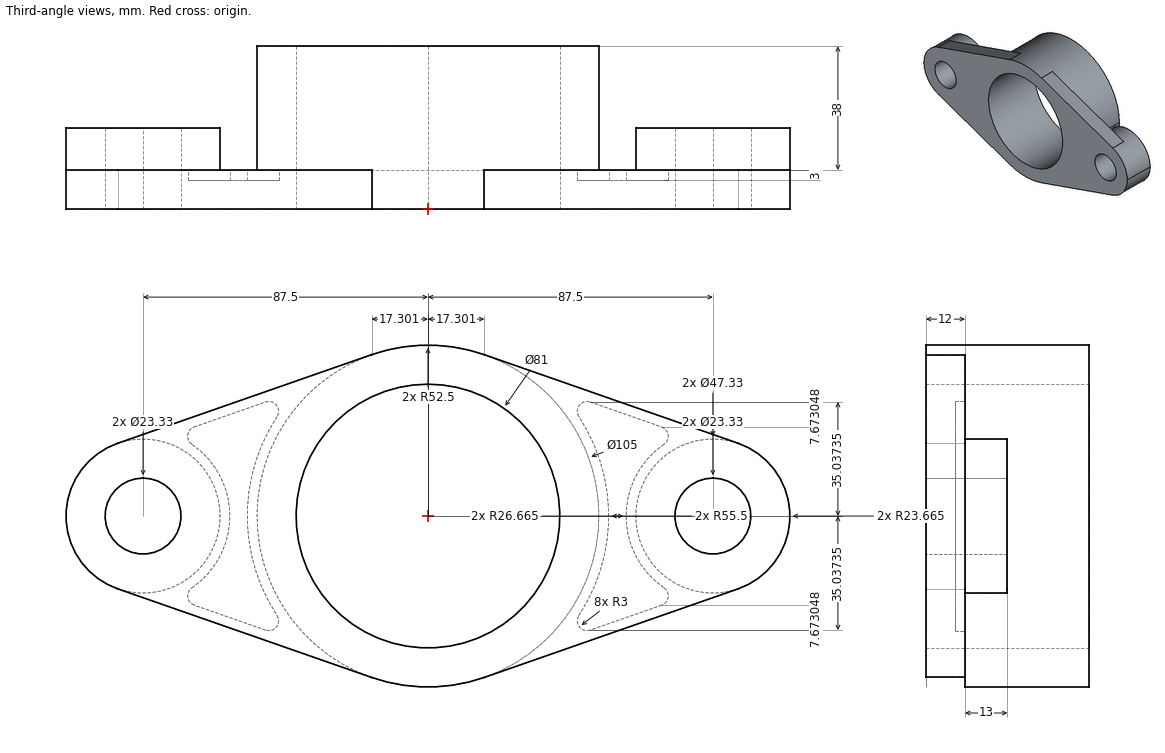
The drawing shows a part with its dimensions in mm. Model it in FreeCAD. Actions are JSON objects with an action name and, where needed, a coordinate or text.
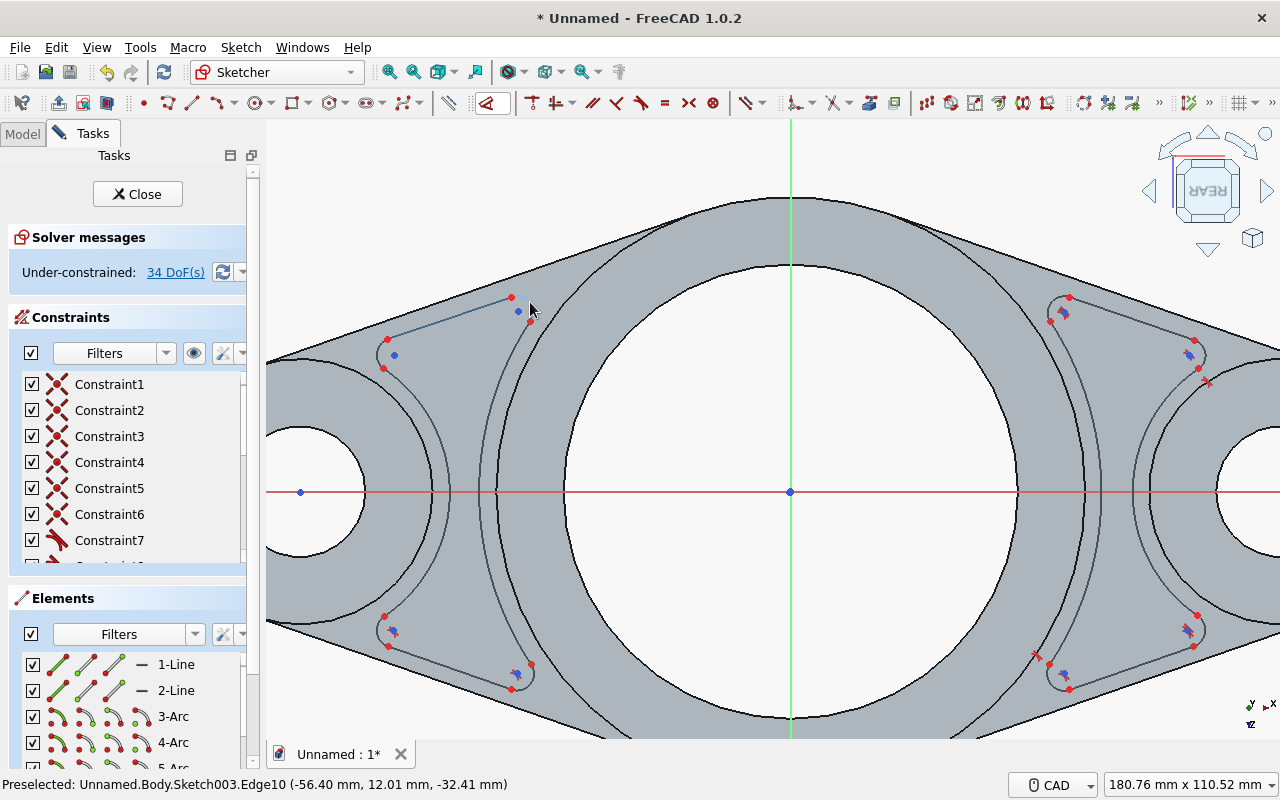
{"action": "left_click", "coordinate": [530, 302]}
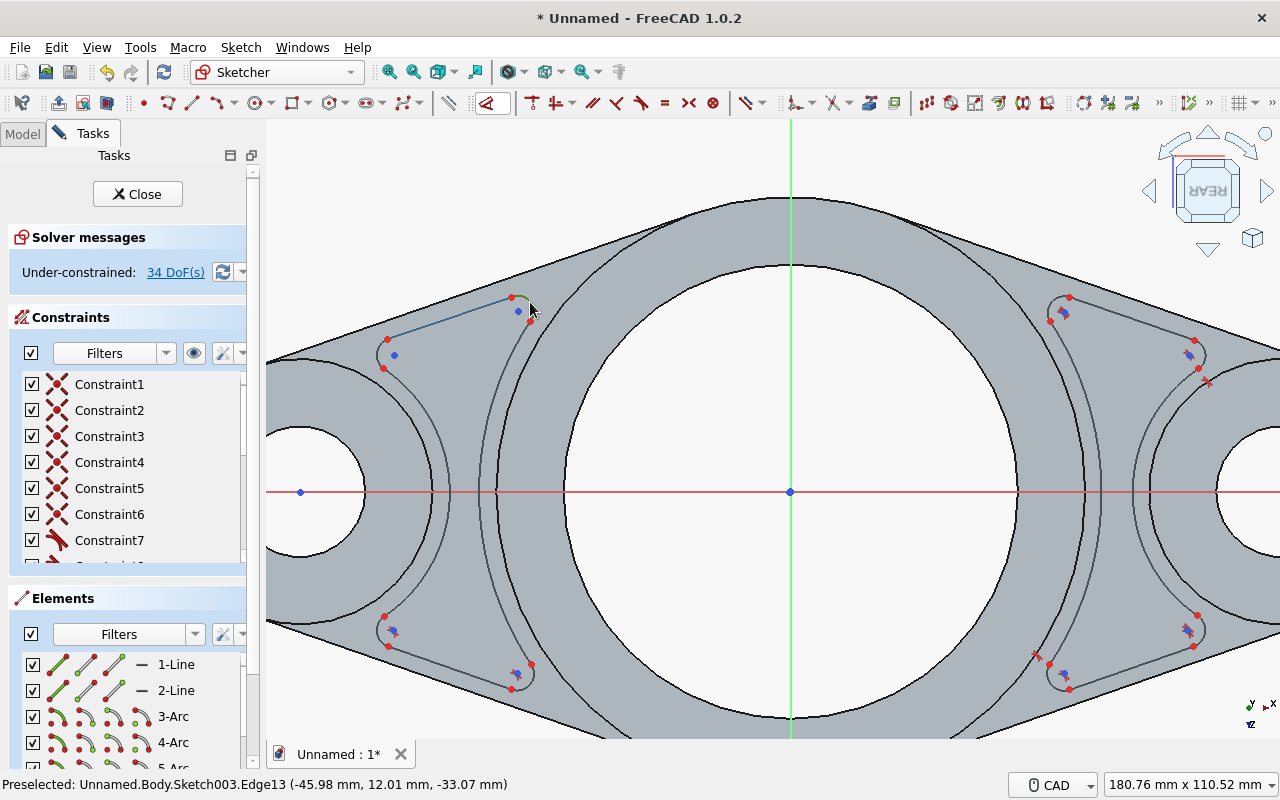
{"action": "left_click", "coordinate": [642, 104]}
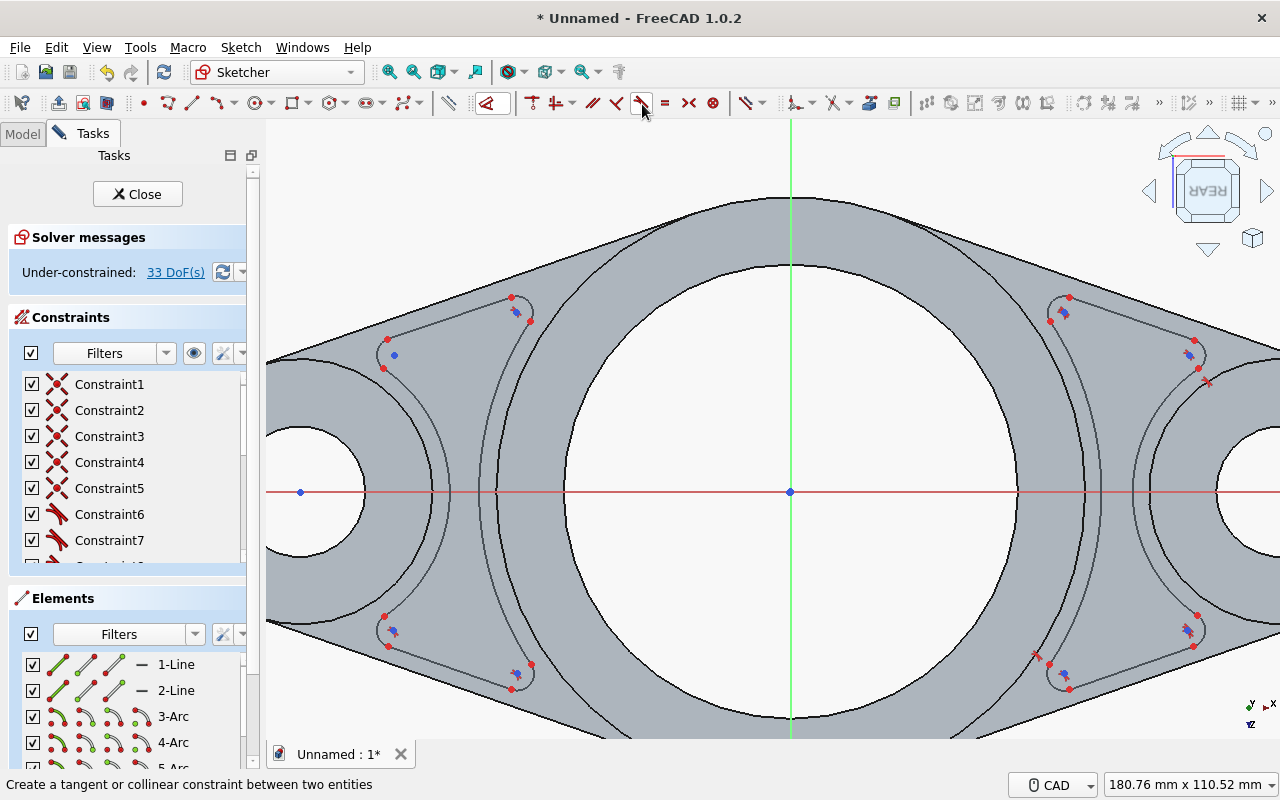
{"action": "left_click", "coordinate": [475, 310]}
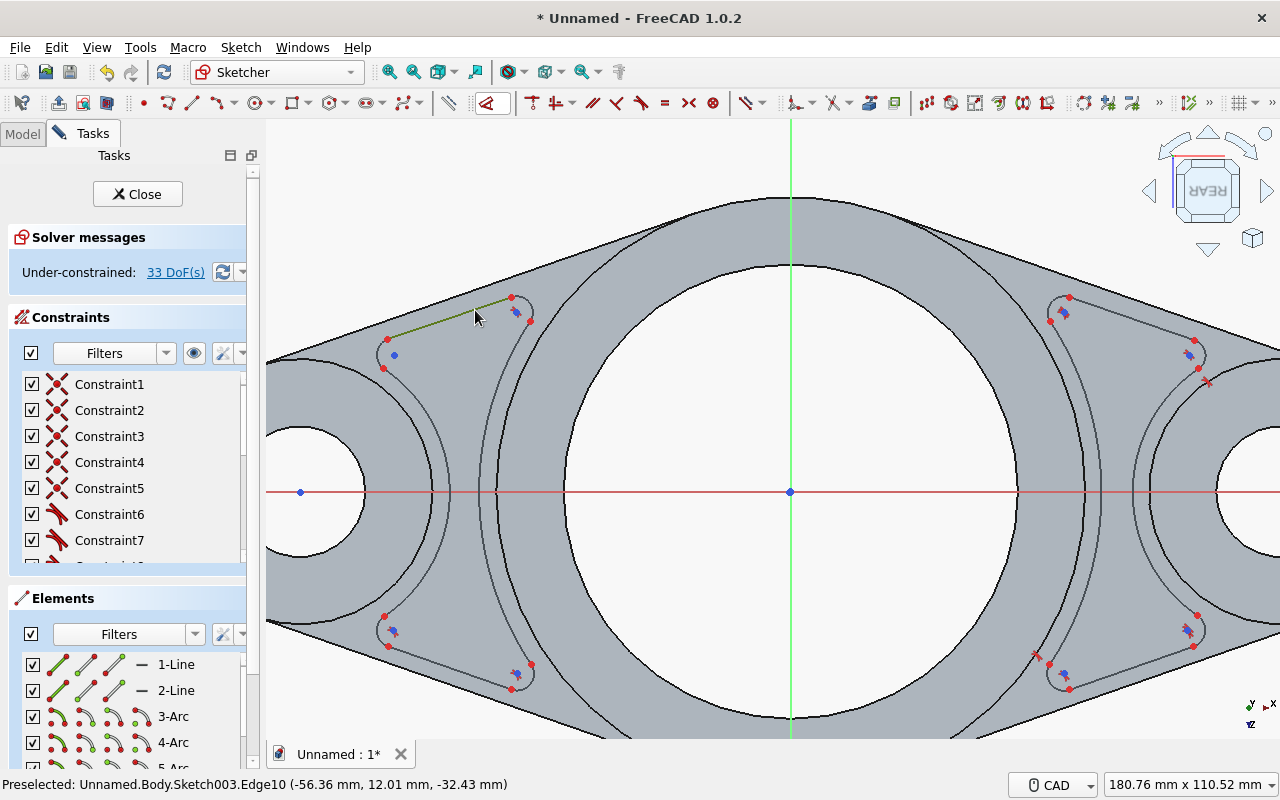
{"action": "scroll", "coordinate": [380, 346], "scroll_direction": "up", "scroll_amount": 2}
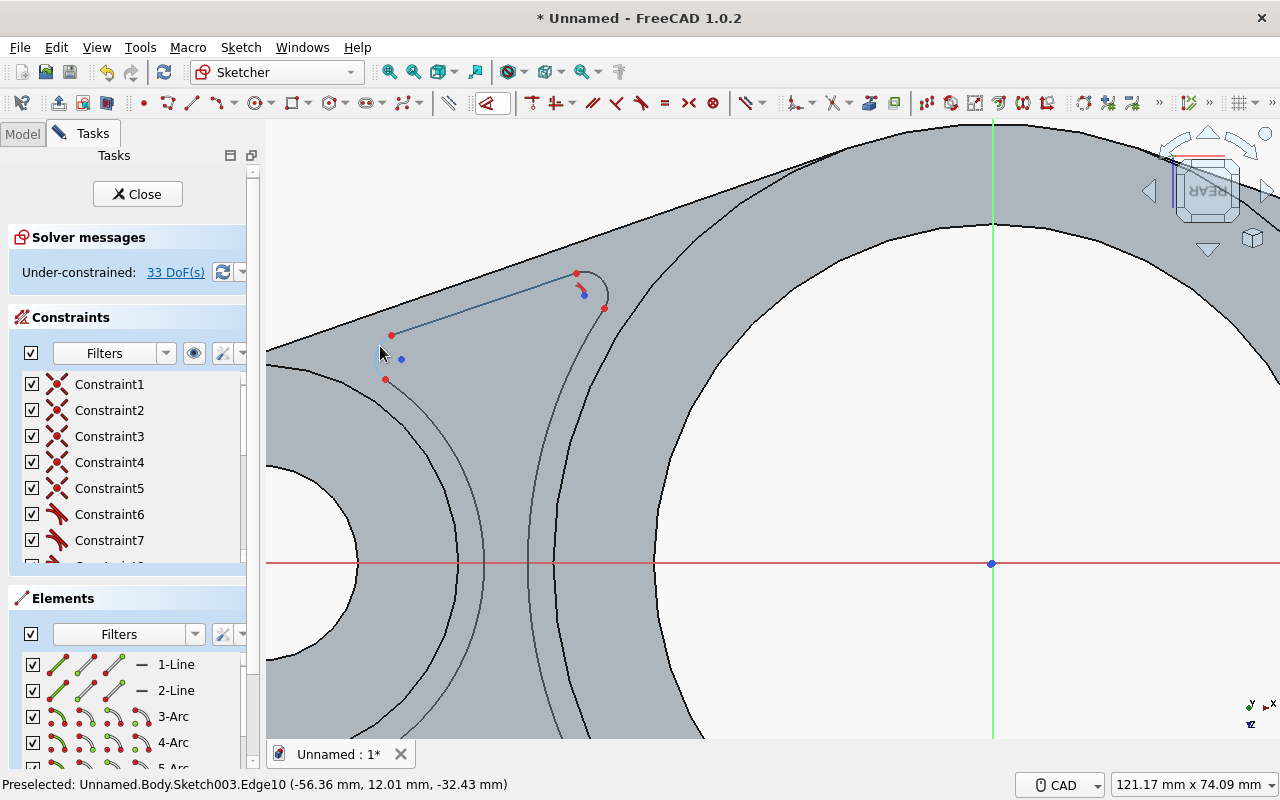
{"action": "left_click", "coordinate": [379, 346]}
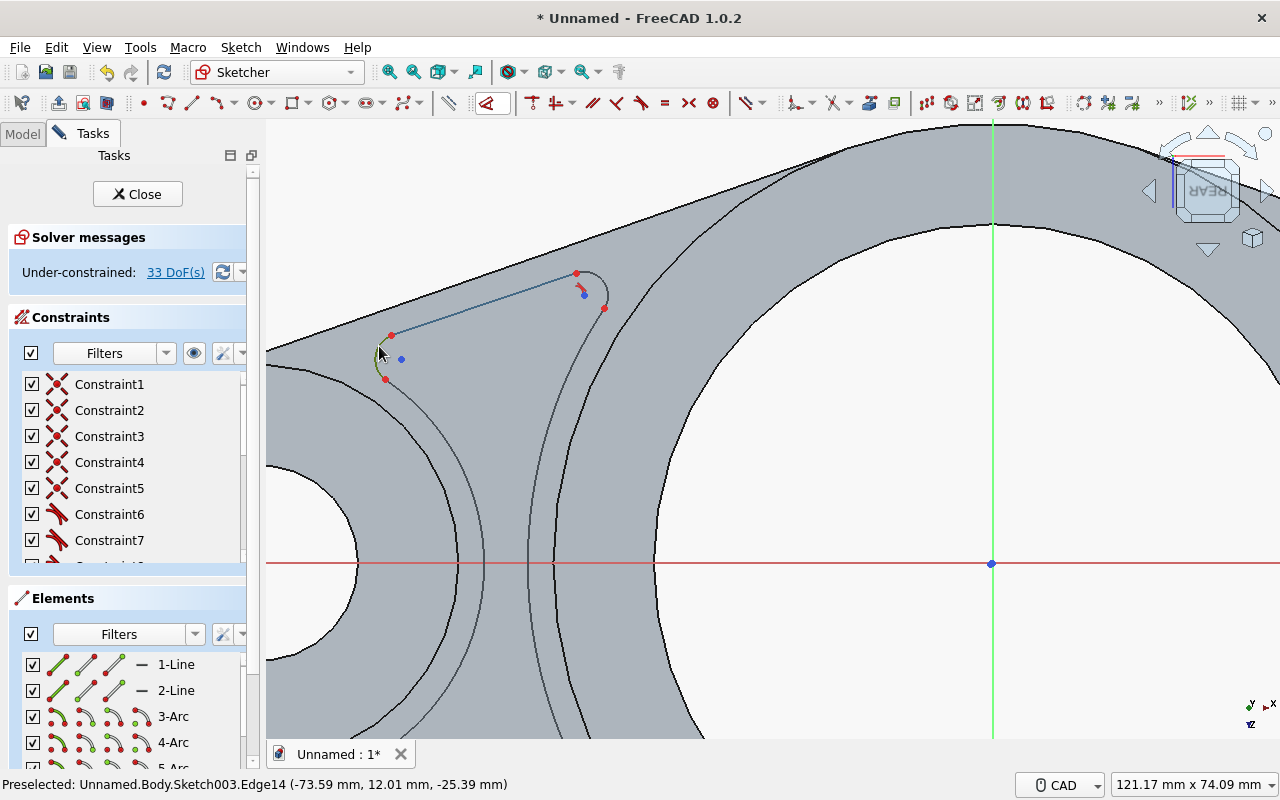
{"action": "left_click", "coordinate": [642, 104]}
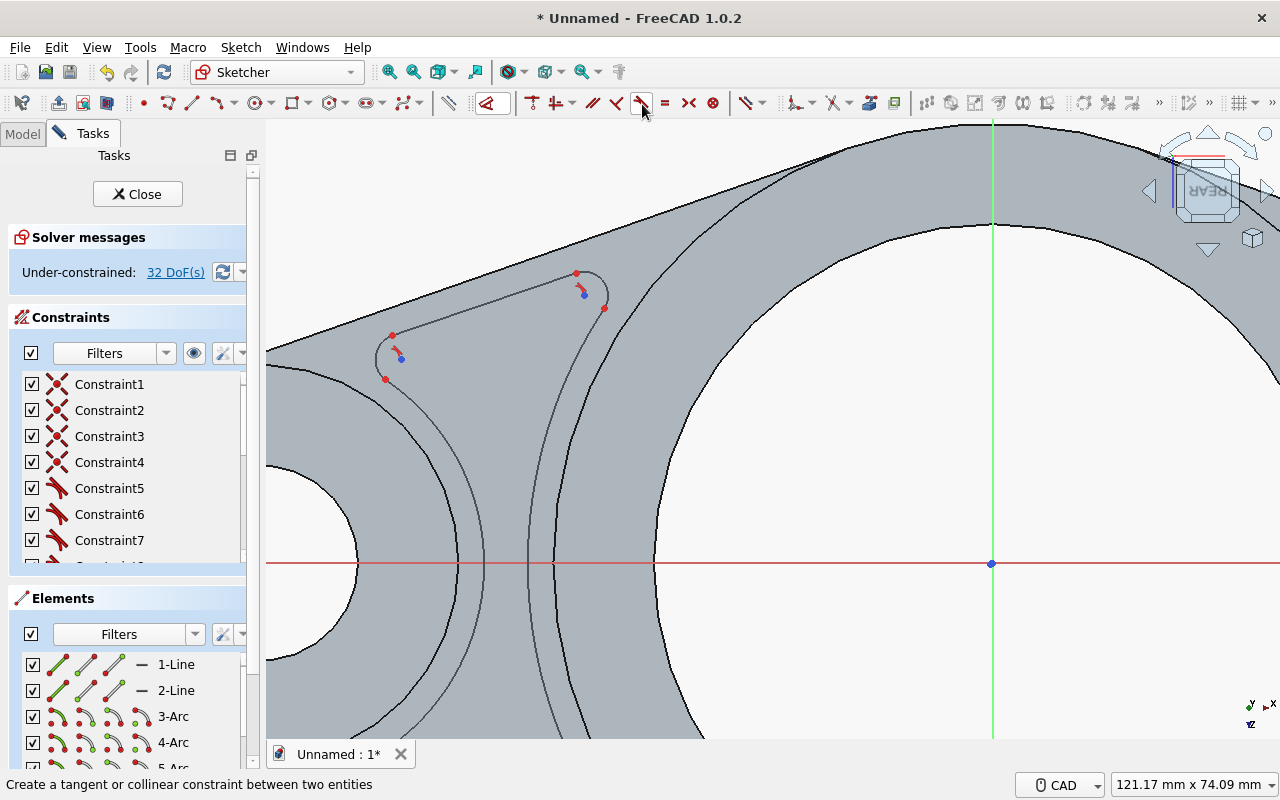
{"action": "scroll", "coordinate": [469, 320], "scroll_direction": "down", "scroll_amount": 4}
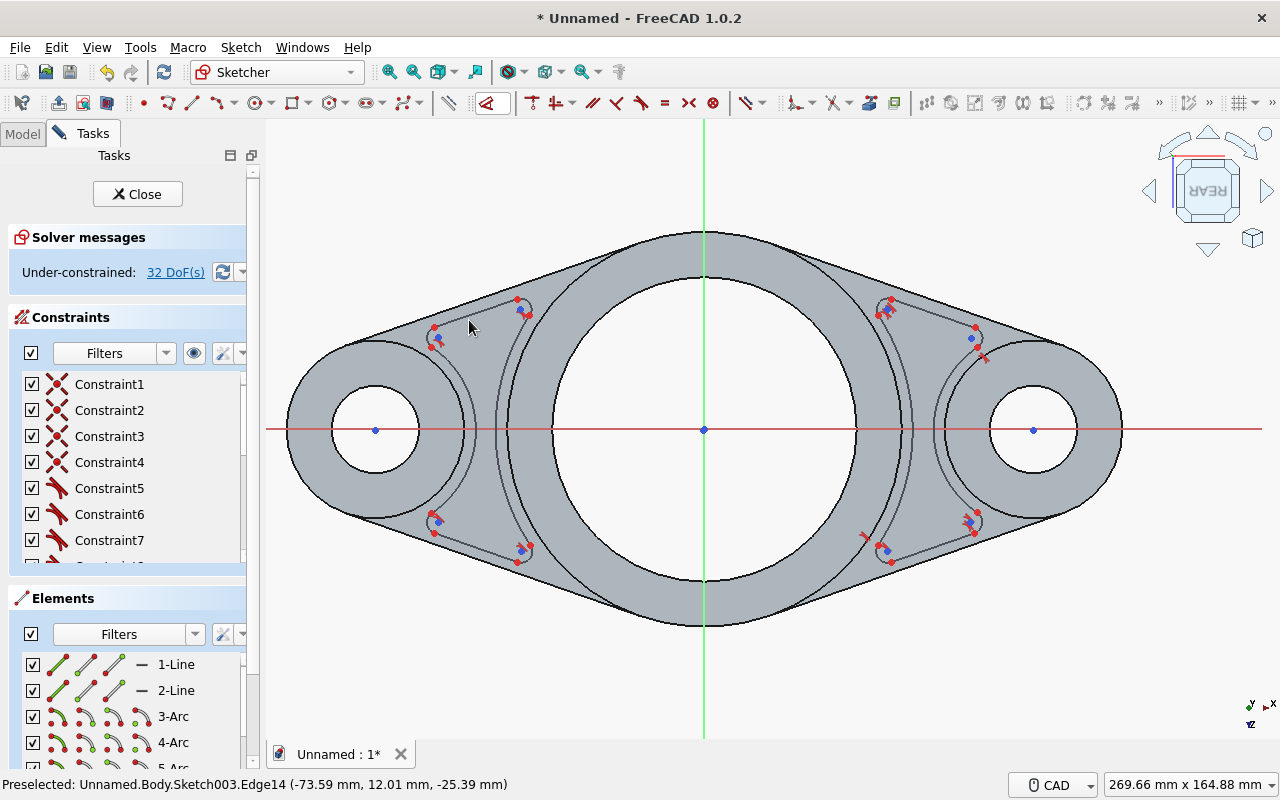
{"action": "scroll", "coordinate": [526, 562], "scroll_direction": "up", "scroll_amount": 3}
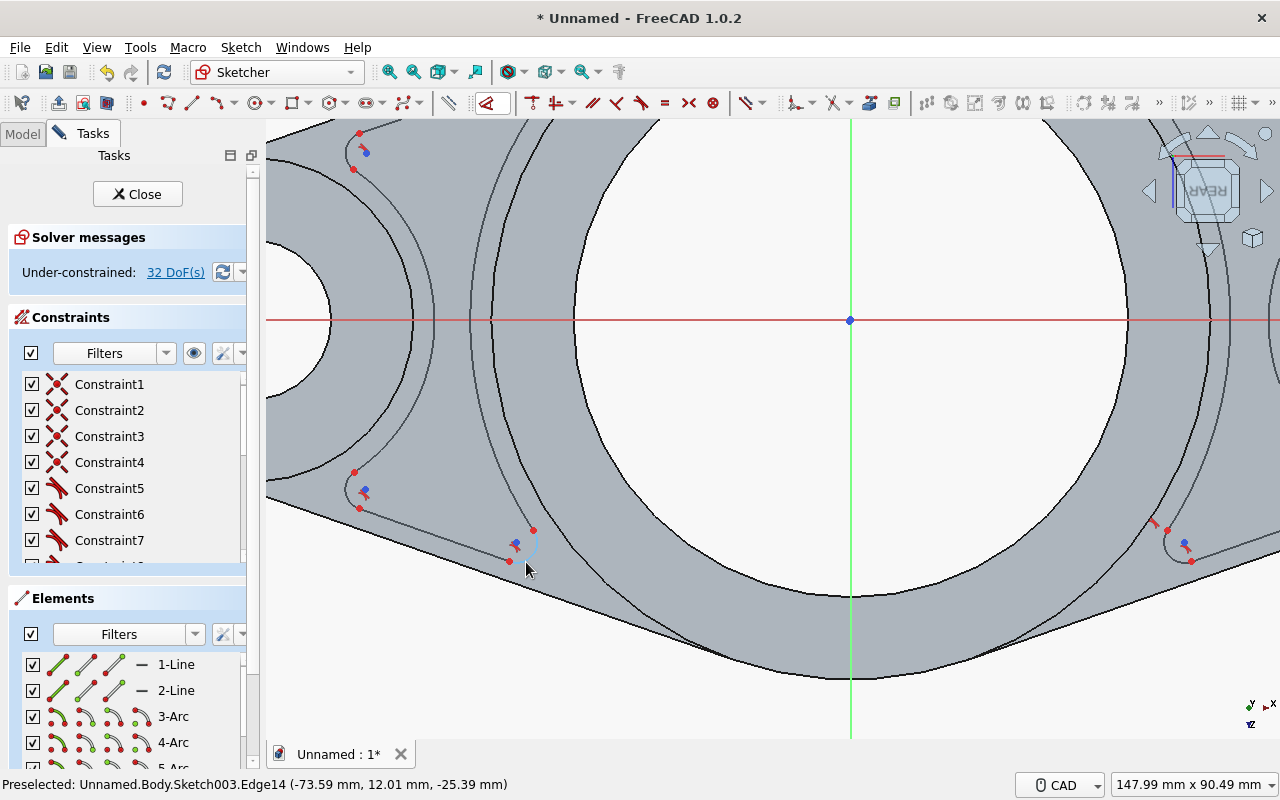
{"action": "left_click", "coordinate": [525, 561]}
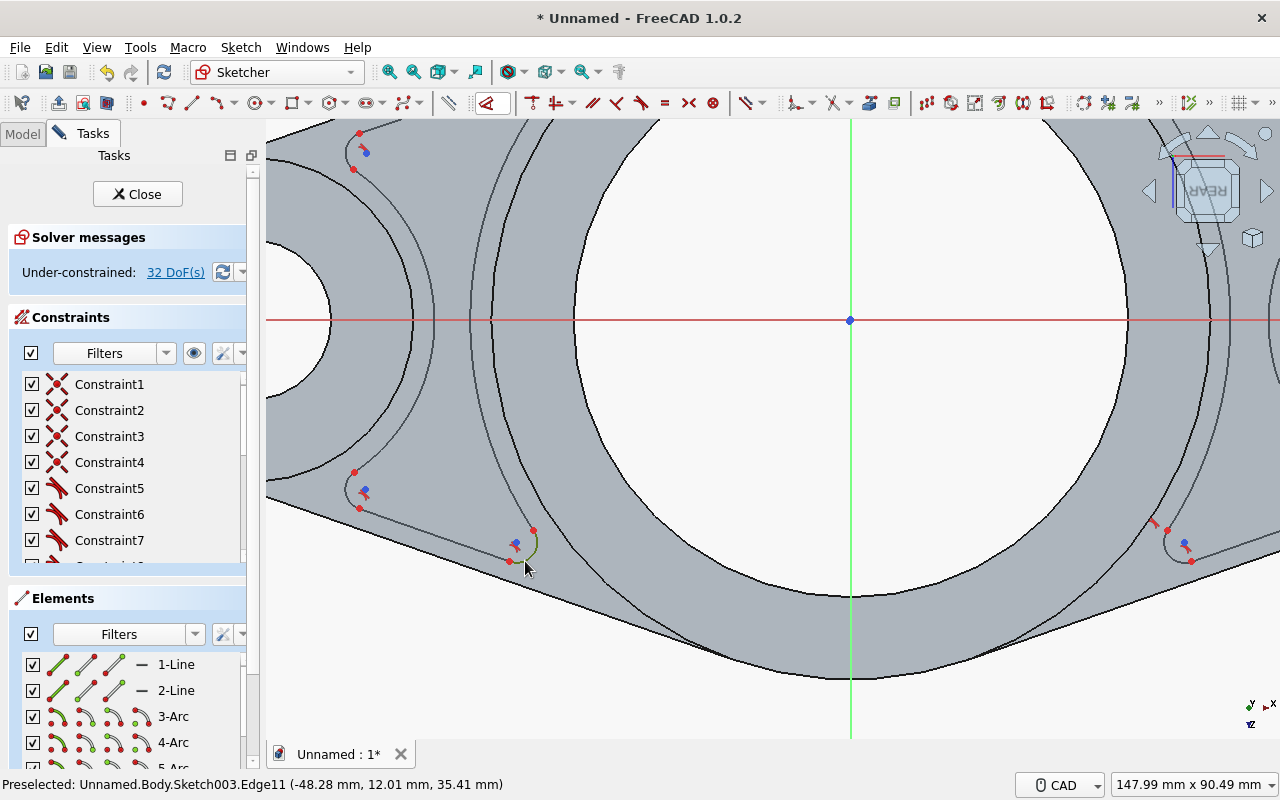
{"action": "left_click", "coordinate": [480, 233]}